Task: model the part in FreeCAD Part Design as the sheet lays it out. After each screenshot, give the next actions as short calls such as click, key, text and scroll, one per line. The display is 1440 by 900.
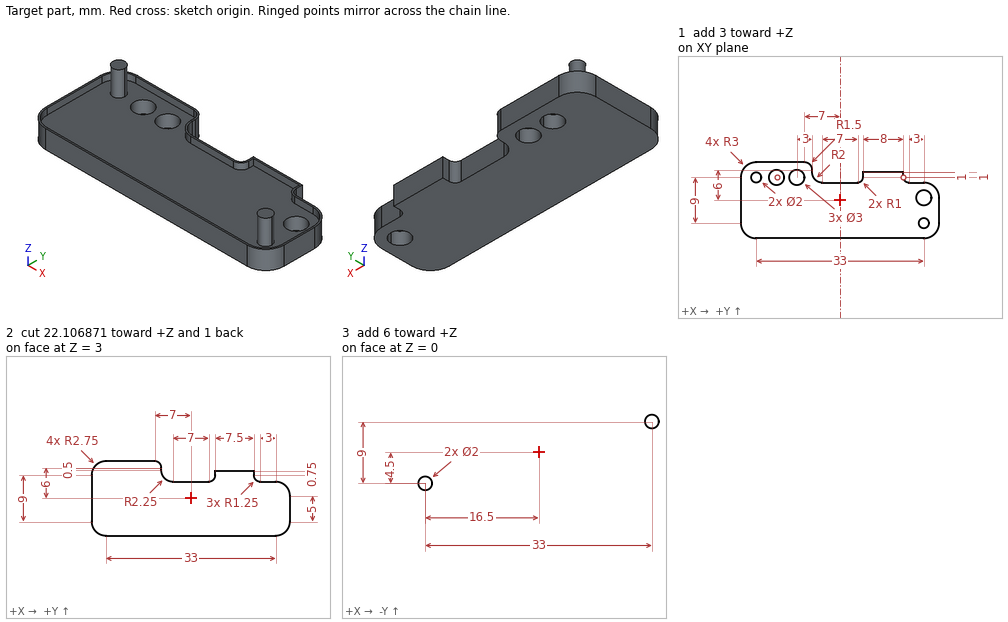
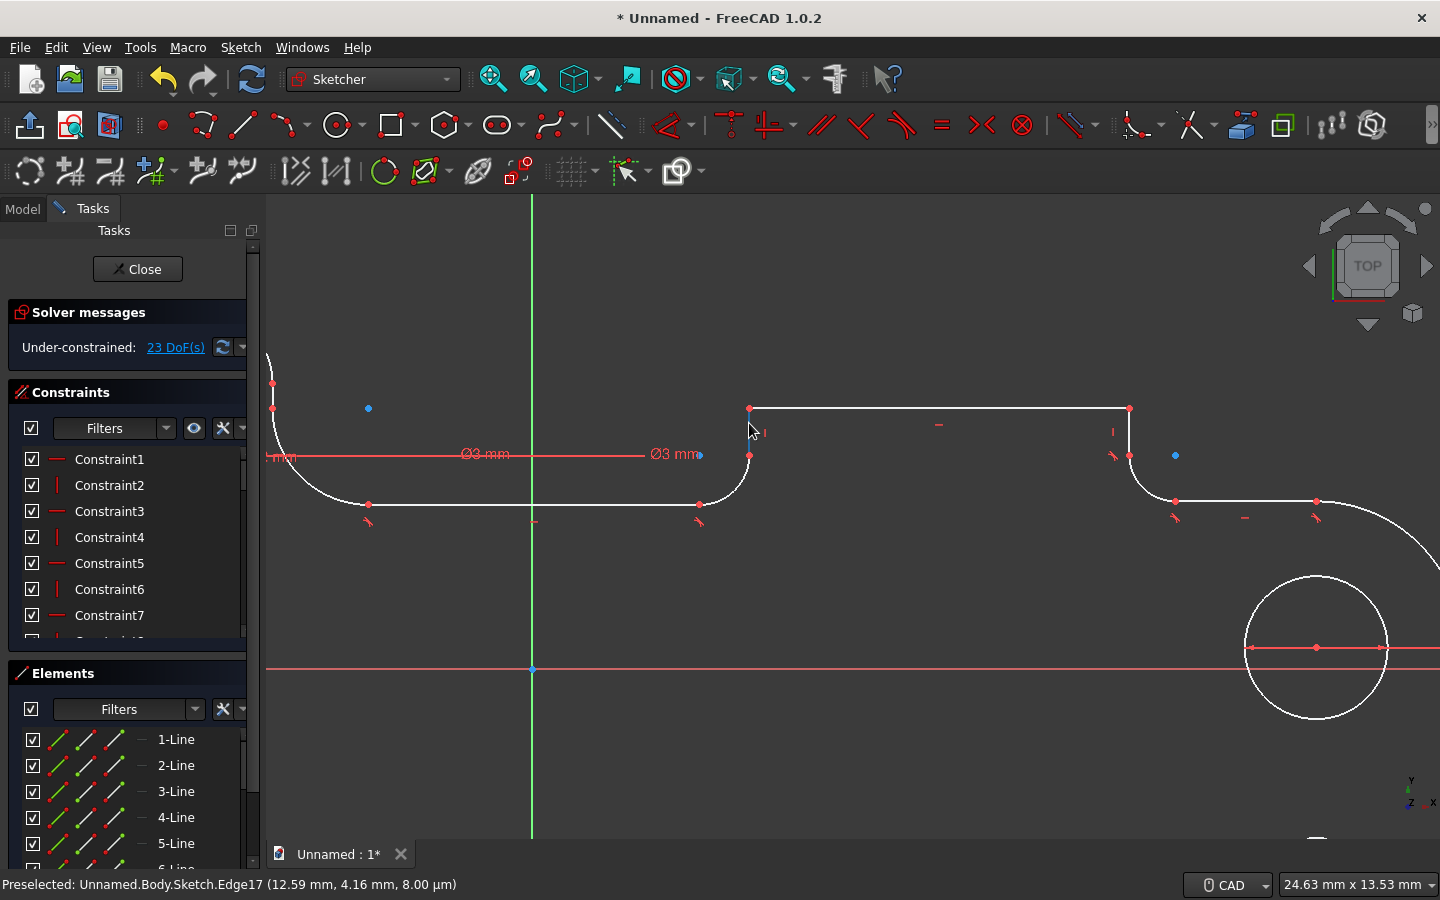
click(749, 423)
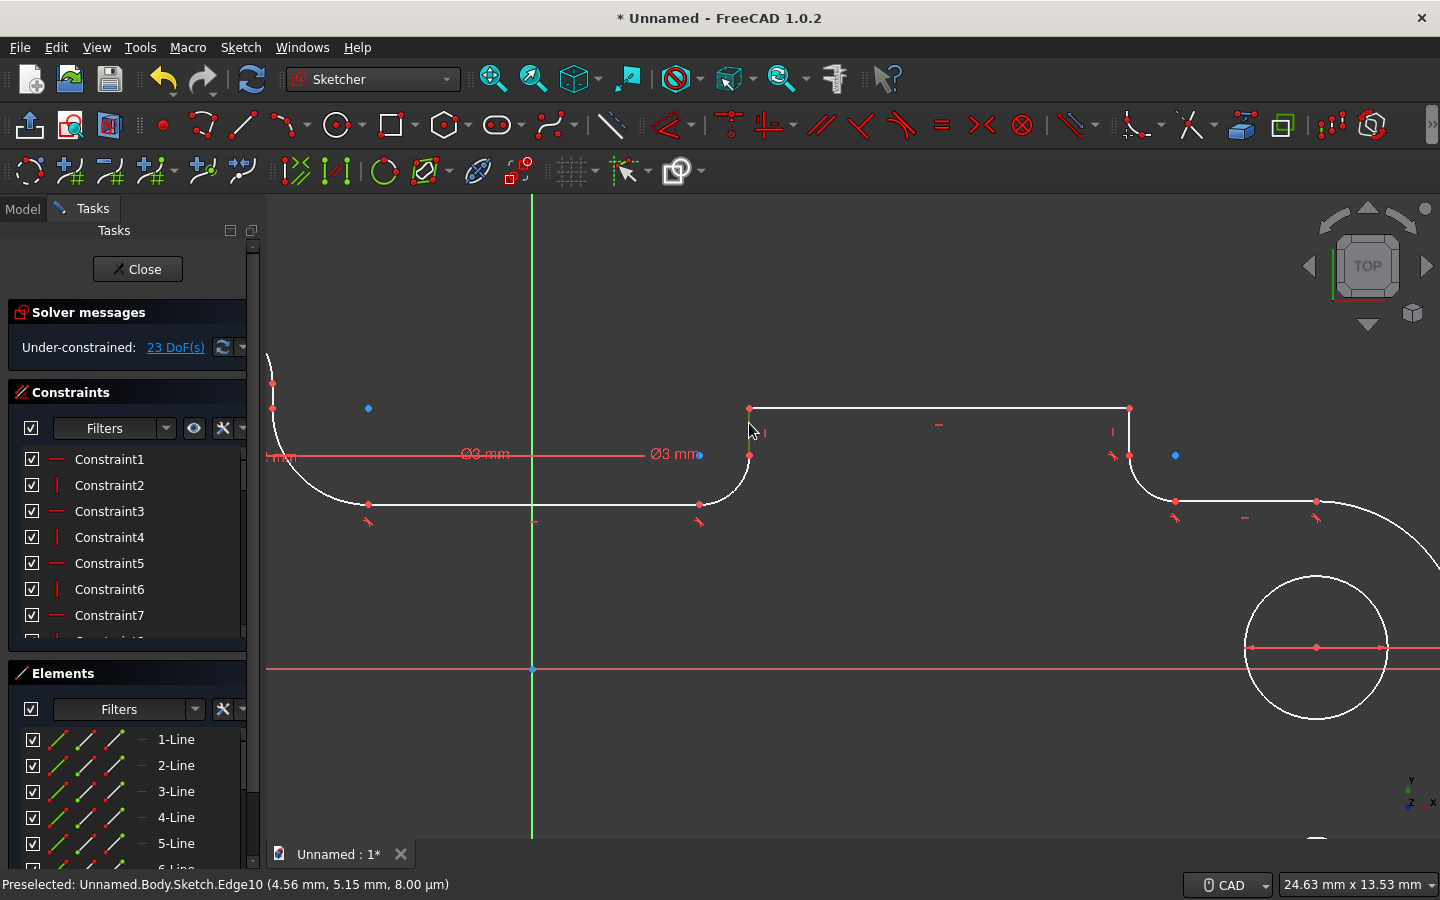
click(722, 500)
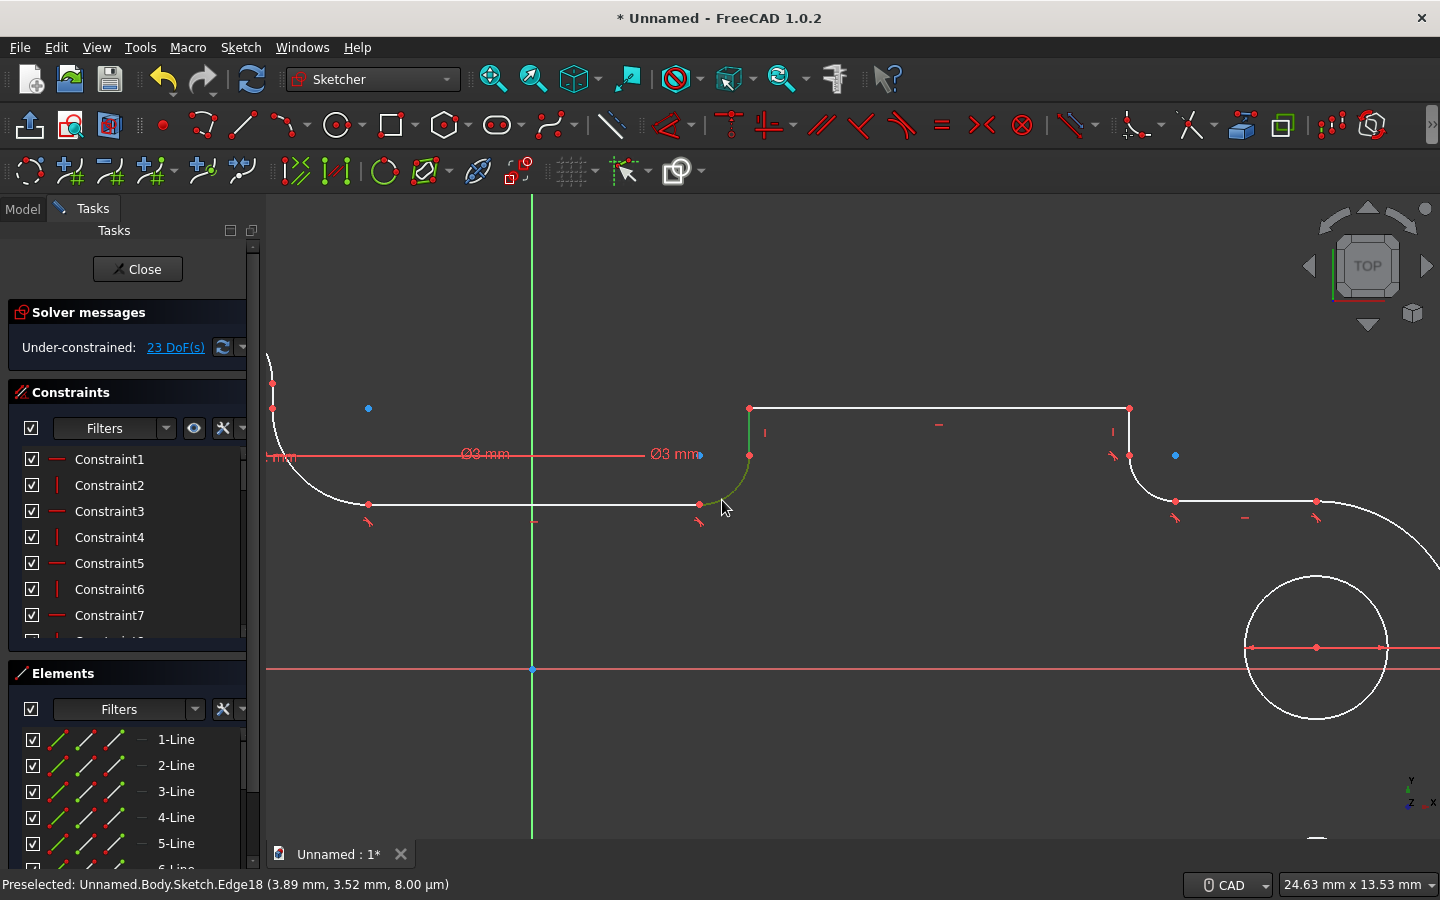
click(902, 126)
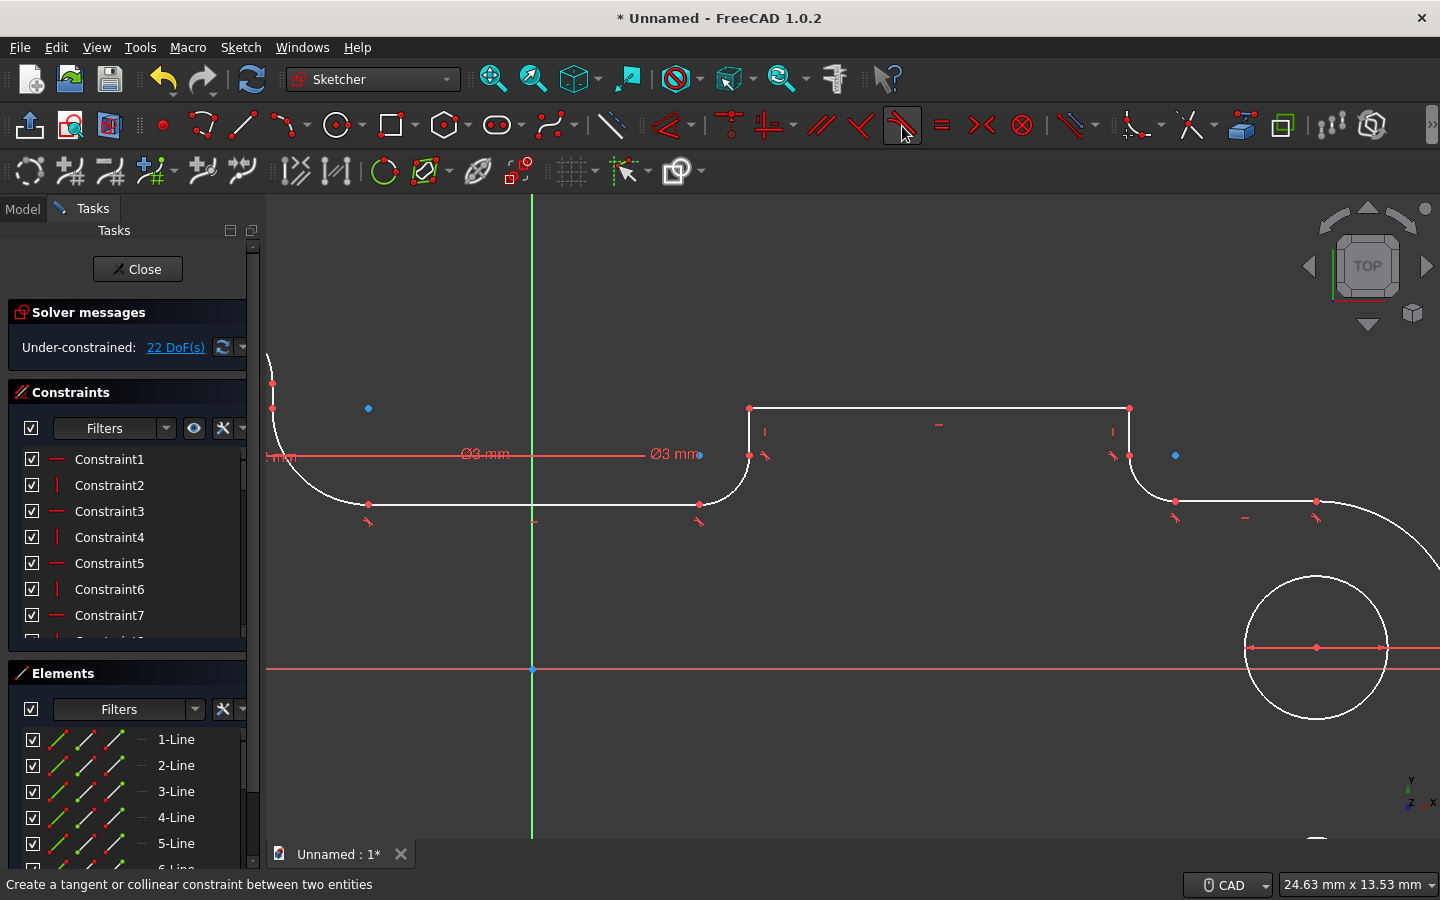
scroll(931, 428, down, 5)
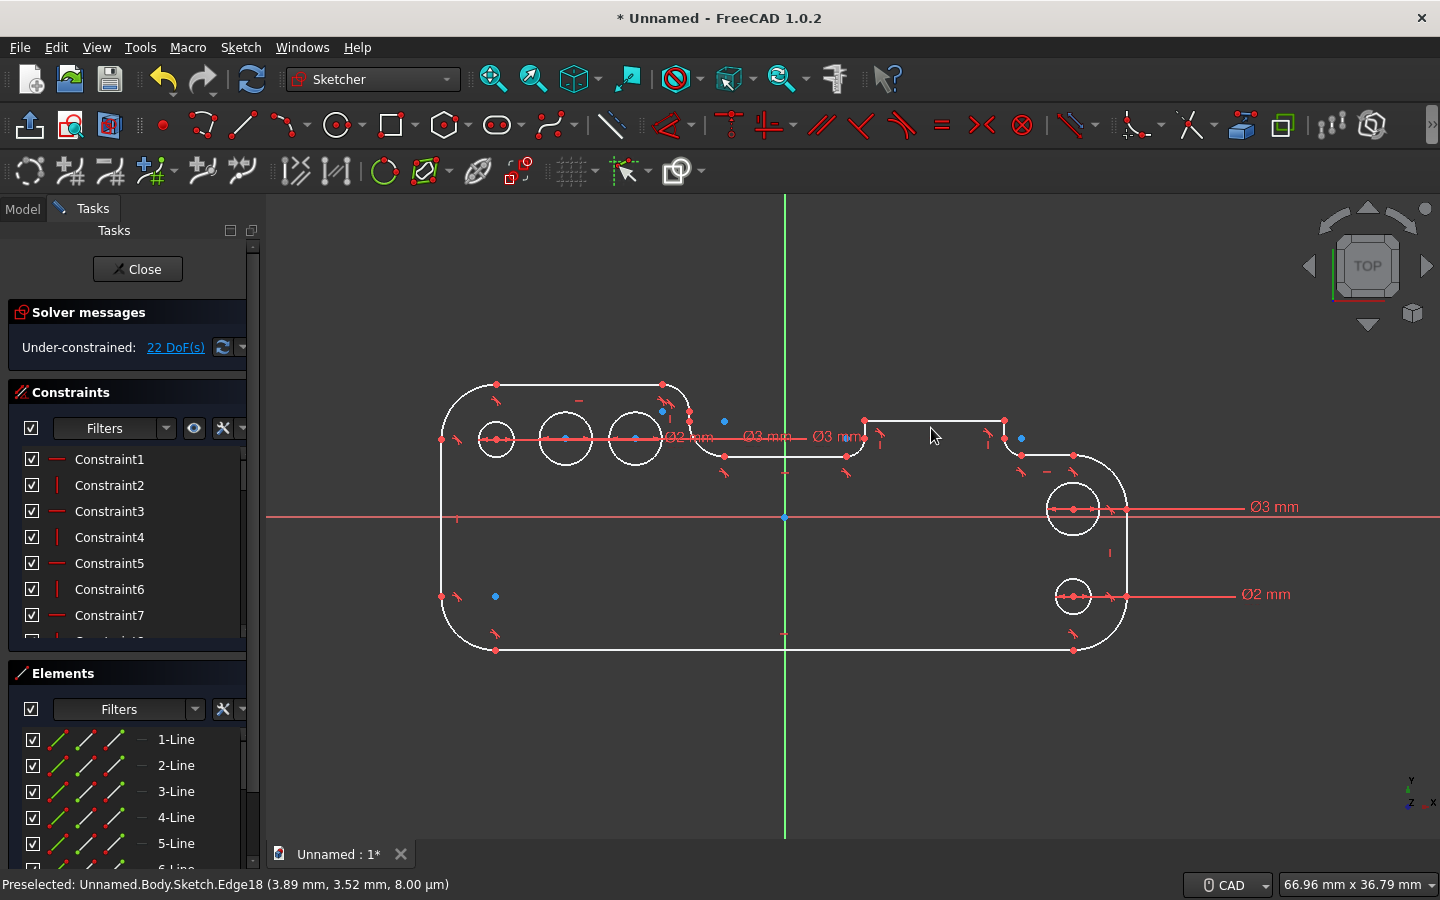
click(471, 391)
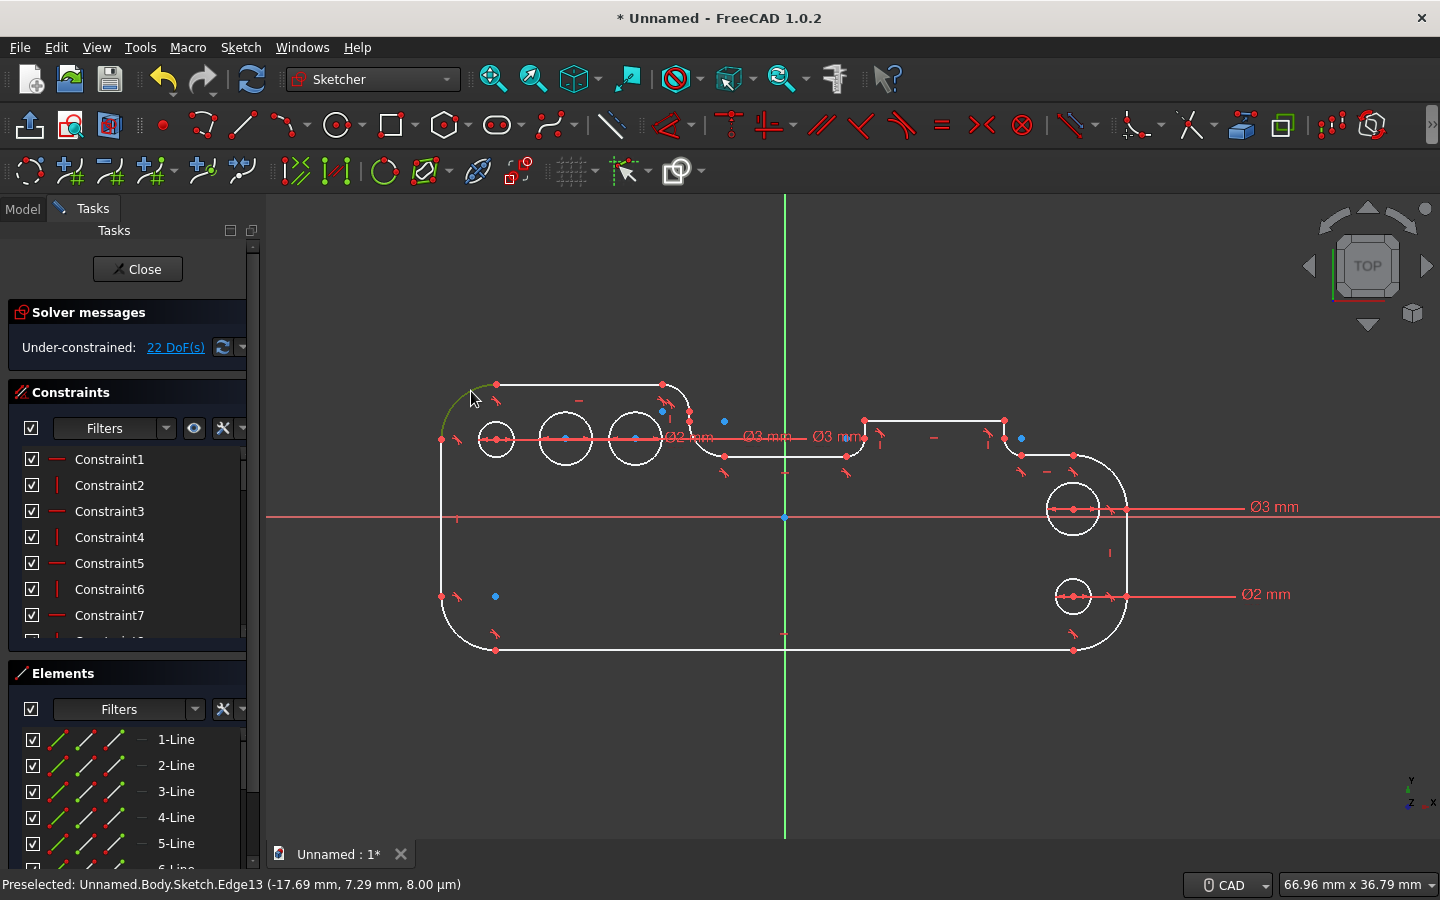
click(447, 621)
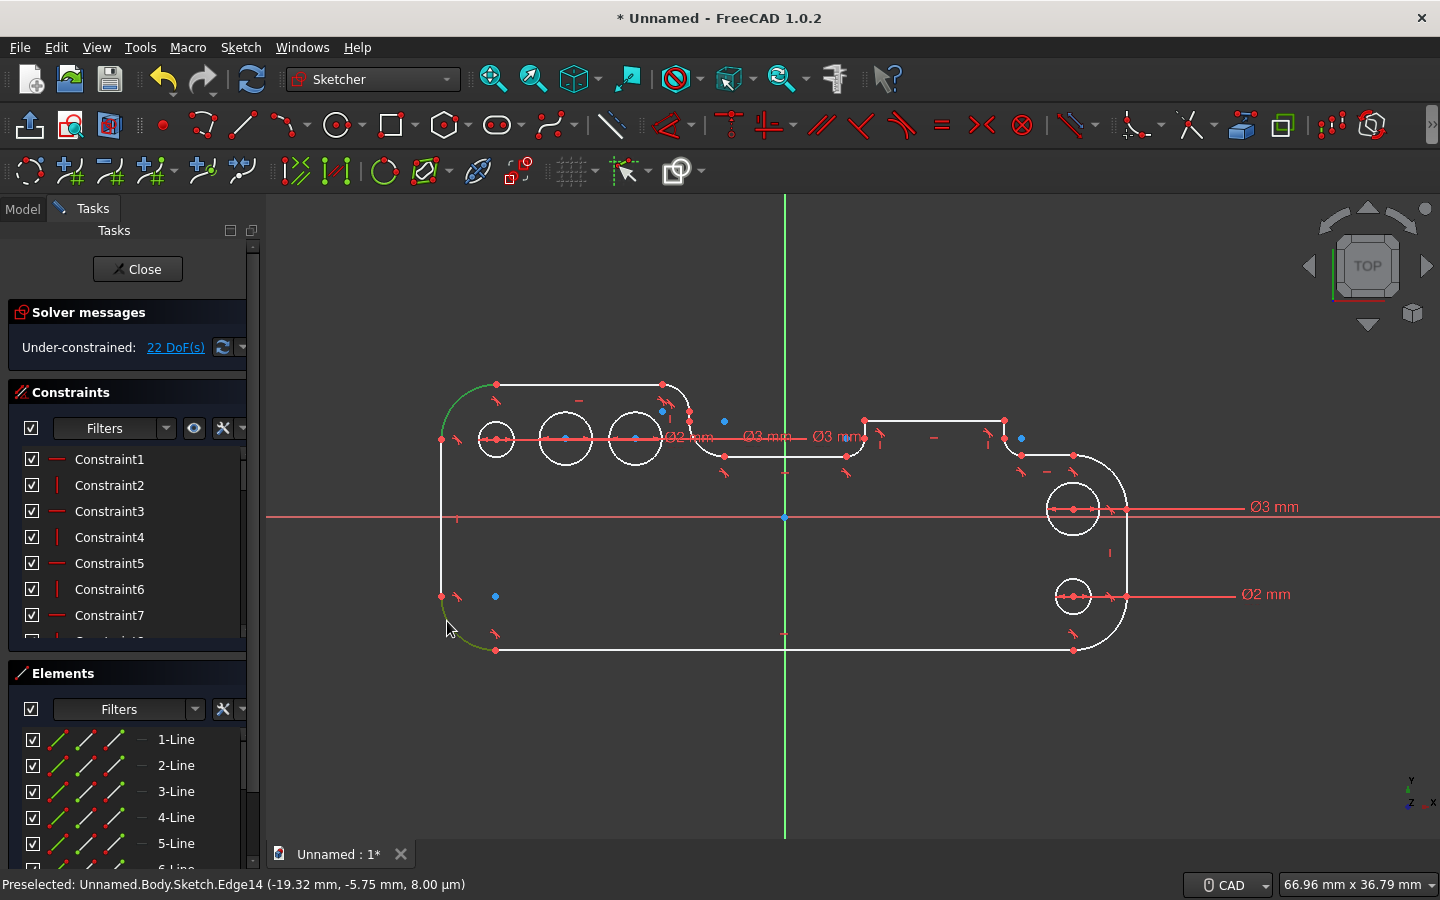
click(1098, 644)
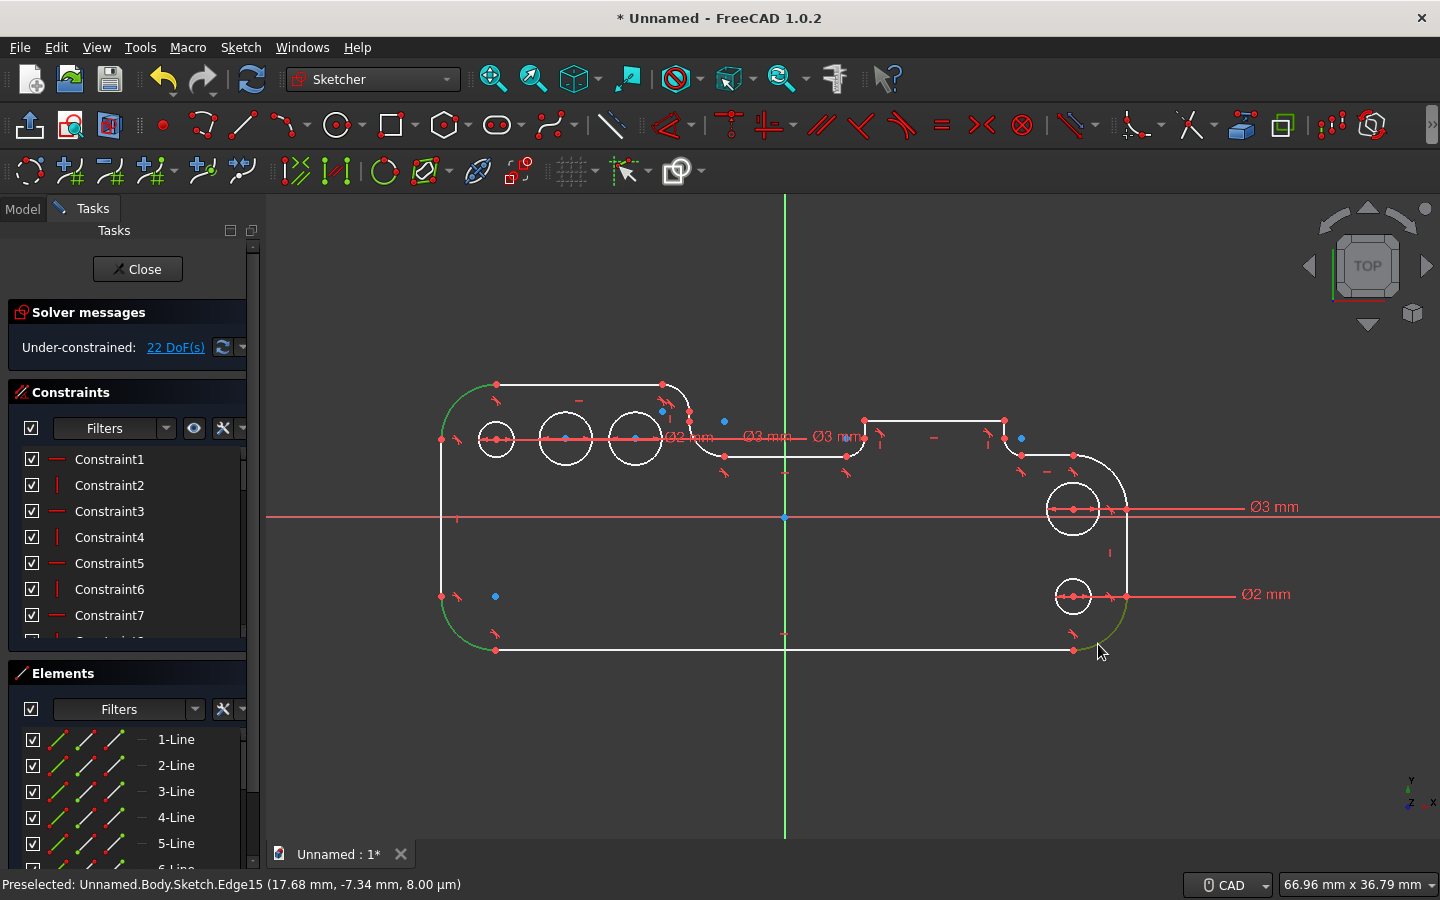
click(1121, 485)